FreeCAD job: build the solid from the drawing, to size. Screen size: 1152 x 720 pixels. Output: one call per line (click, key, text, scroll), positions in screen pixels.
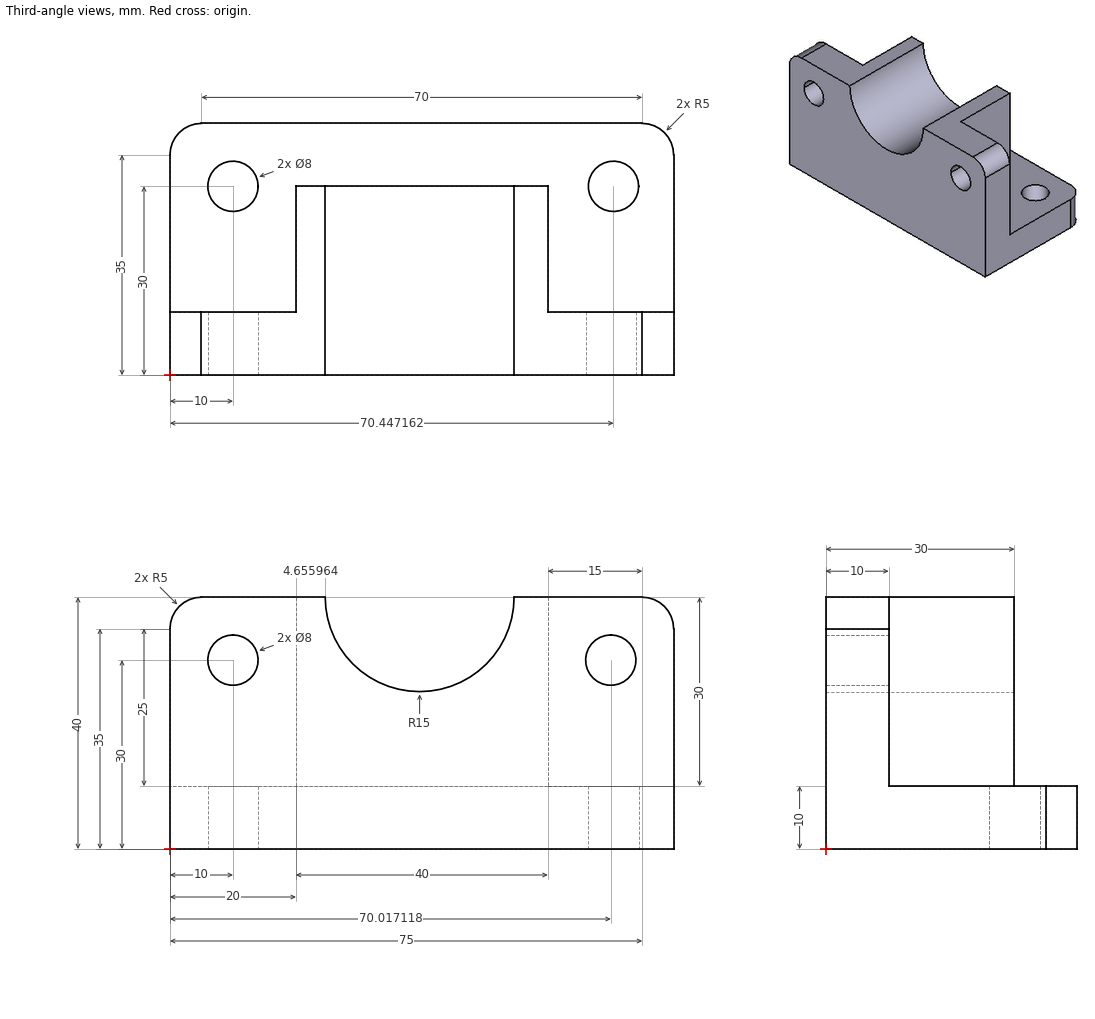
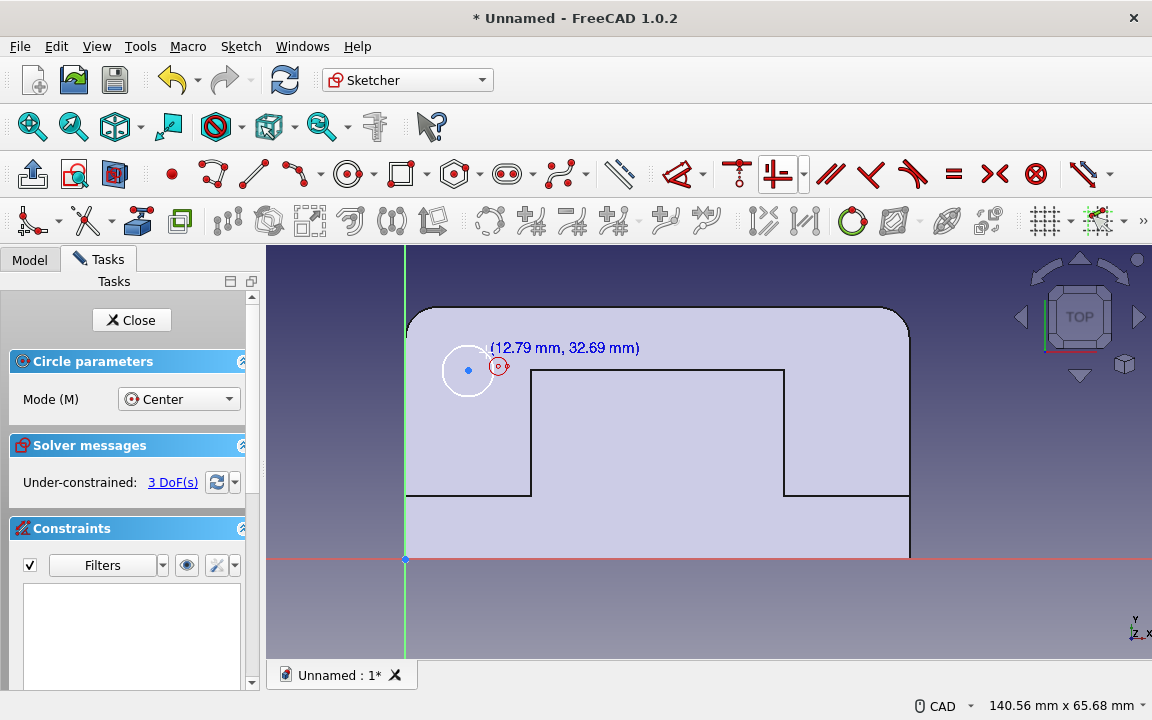
click(849, 370)
click(867, 352)
key(Escape)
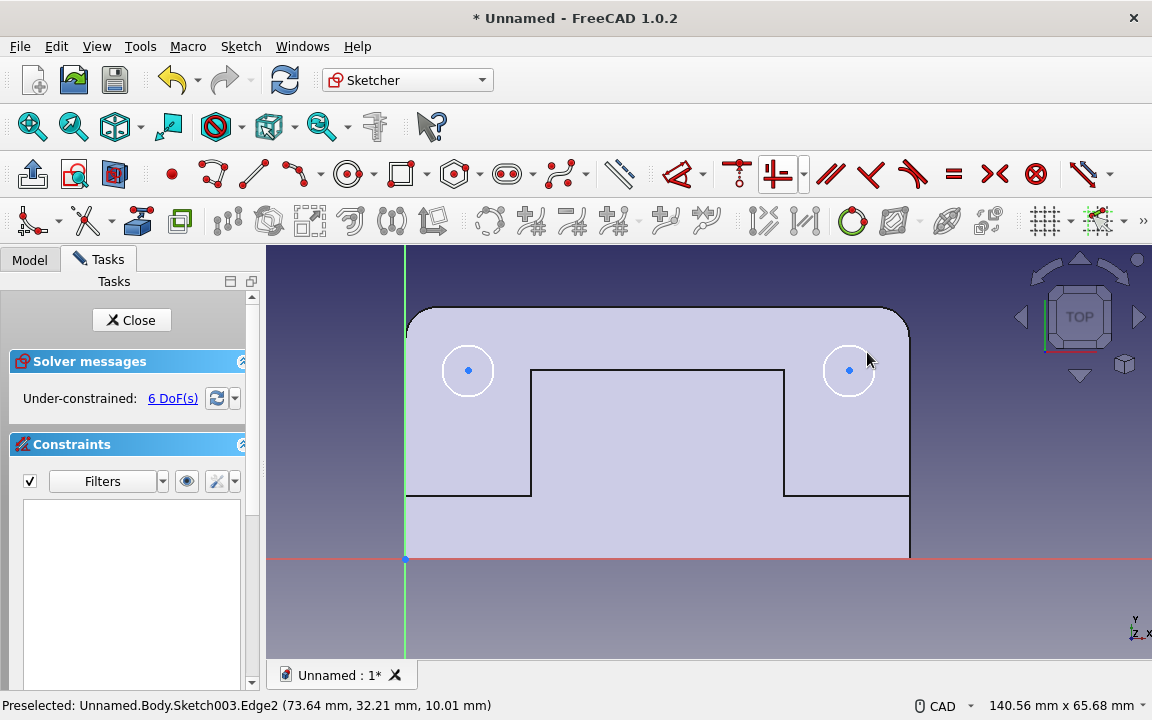
click(486, 353)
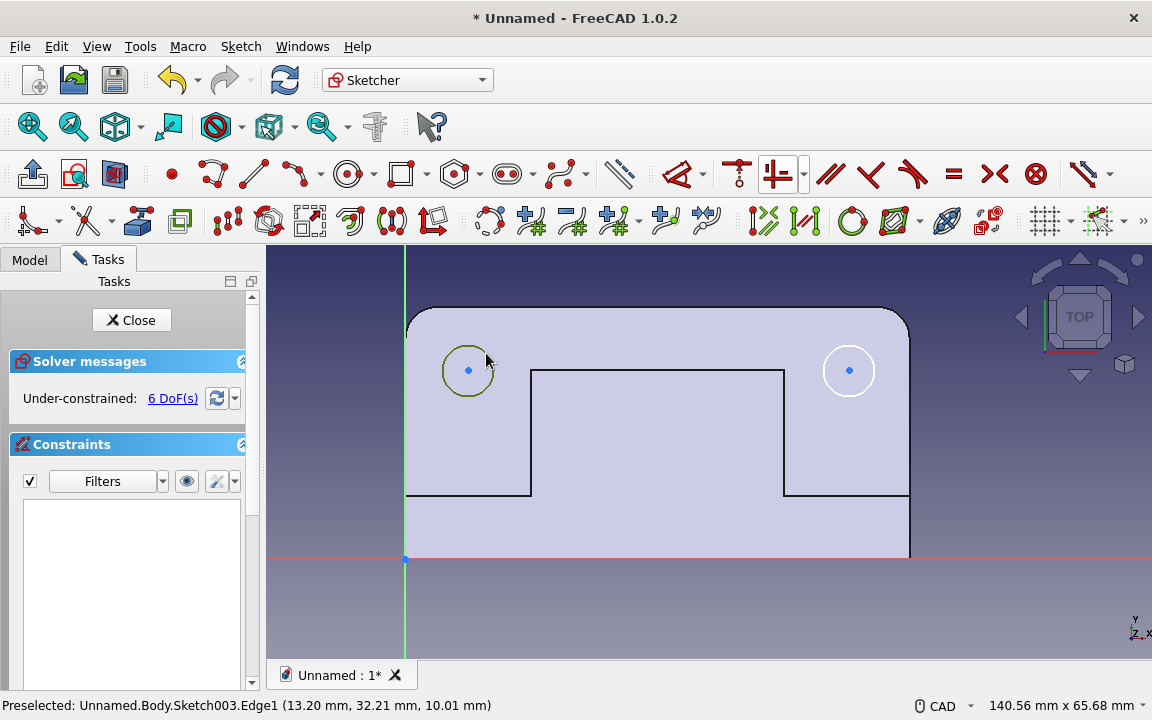
click(867, 353)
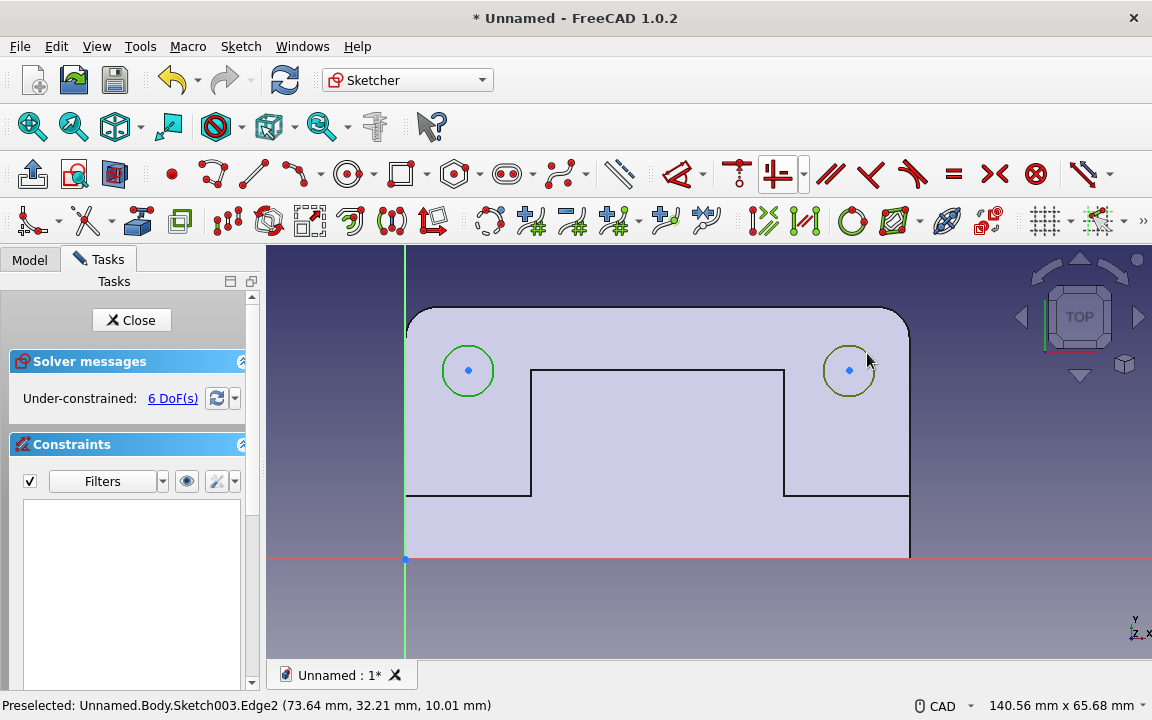
click(954, 174)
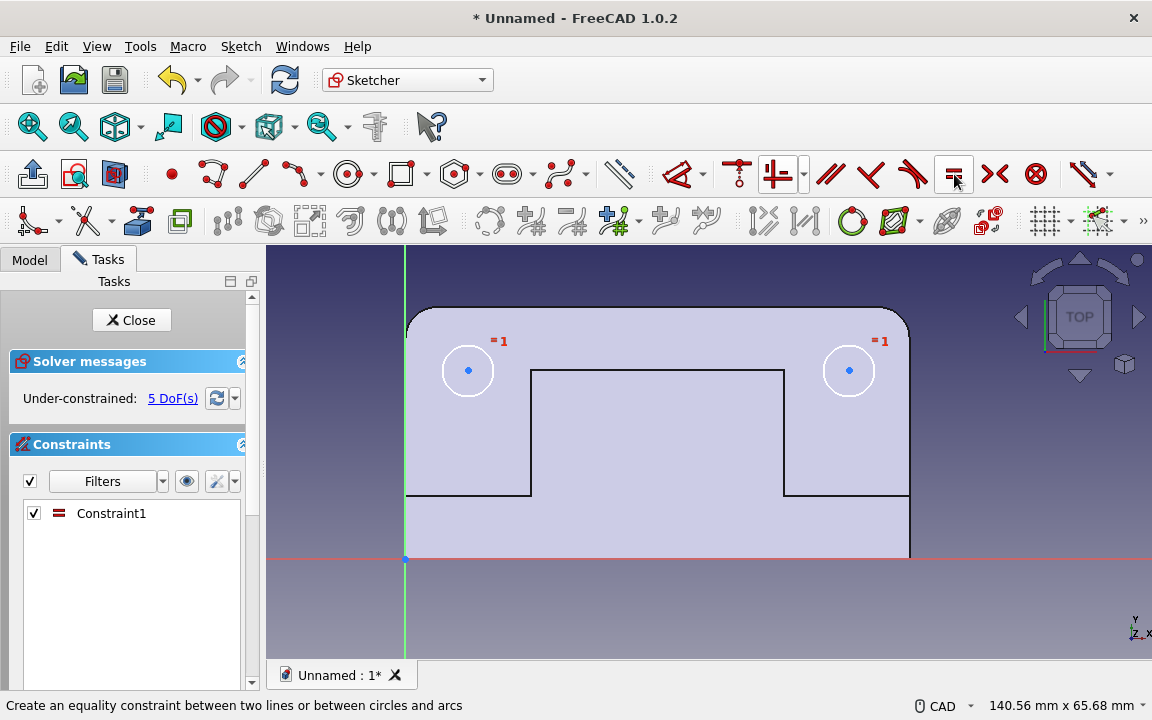
click(468, 371)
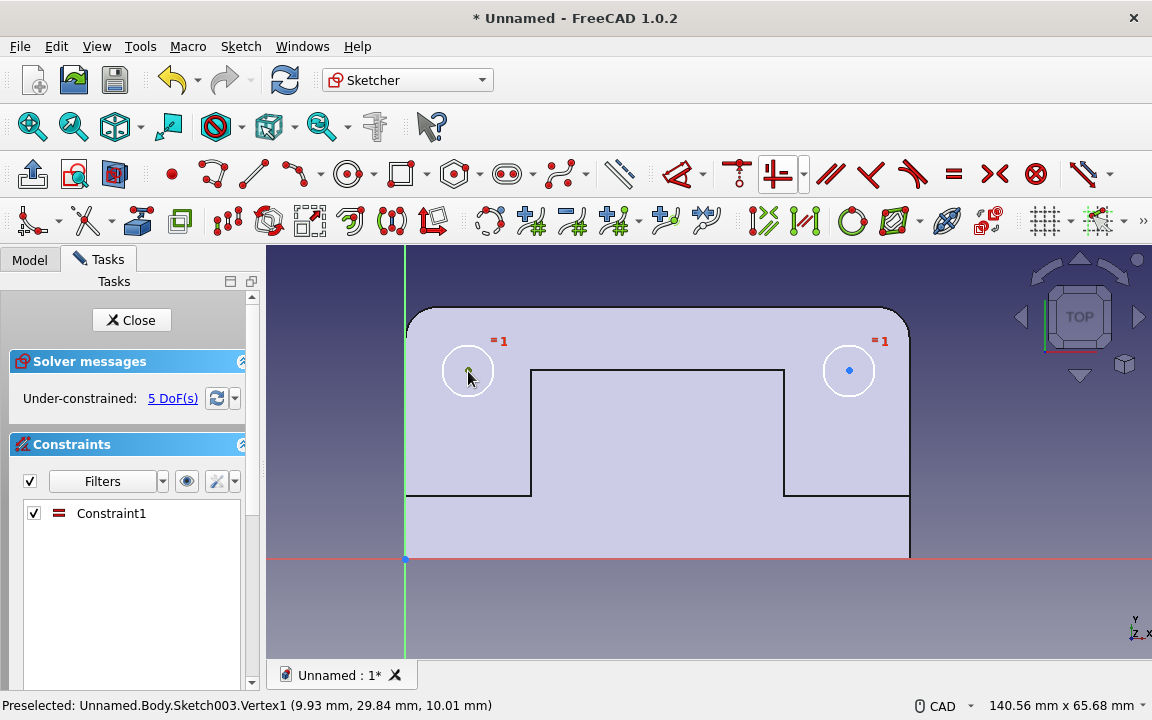
click(849, 371)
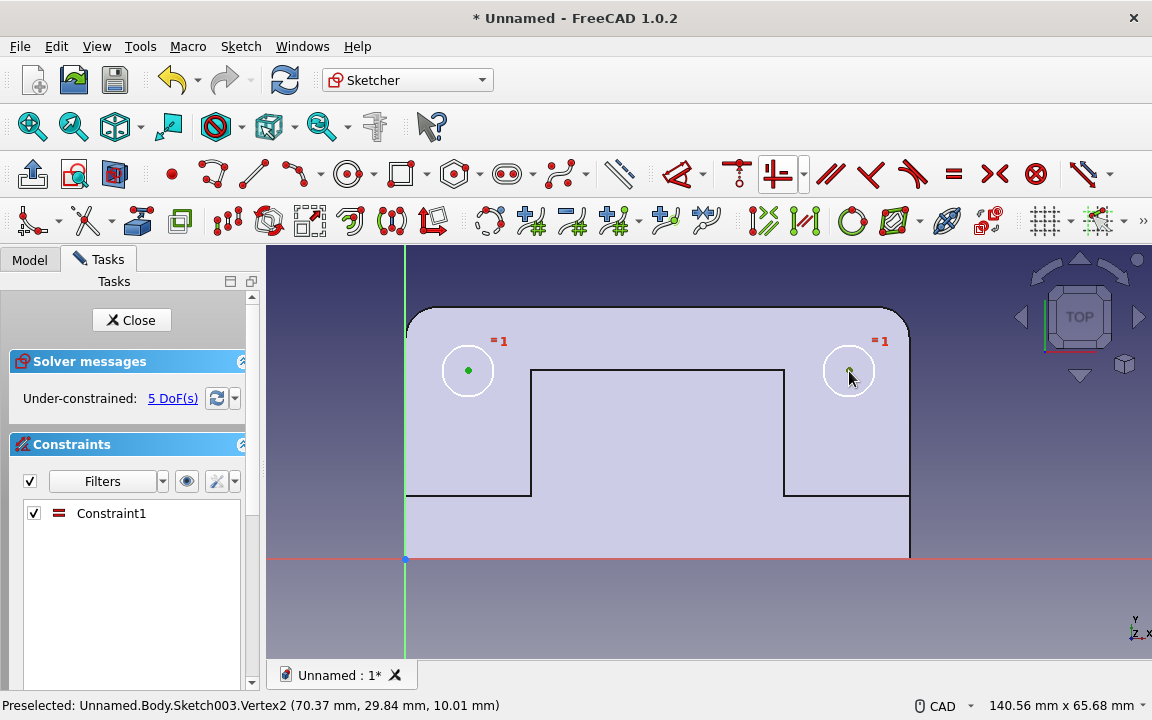
key(h)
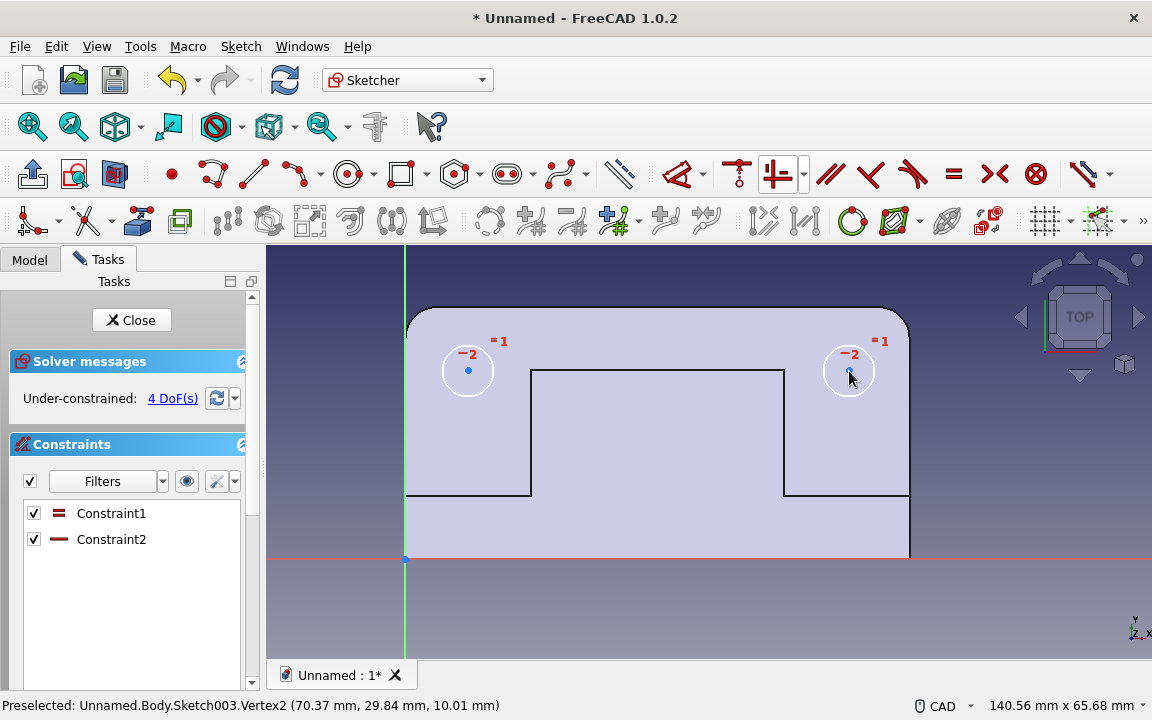
click(676, 174)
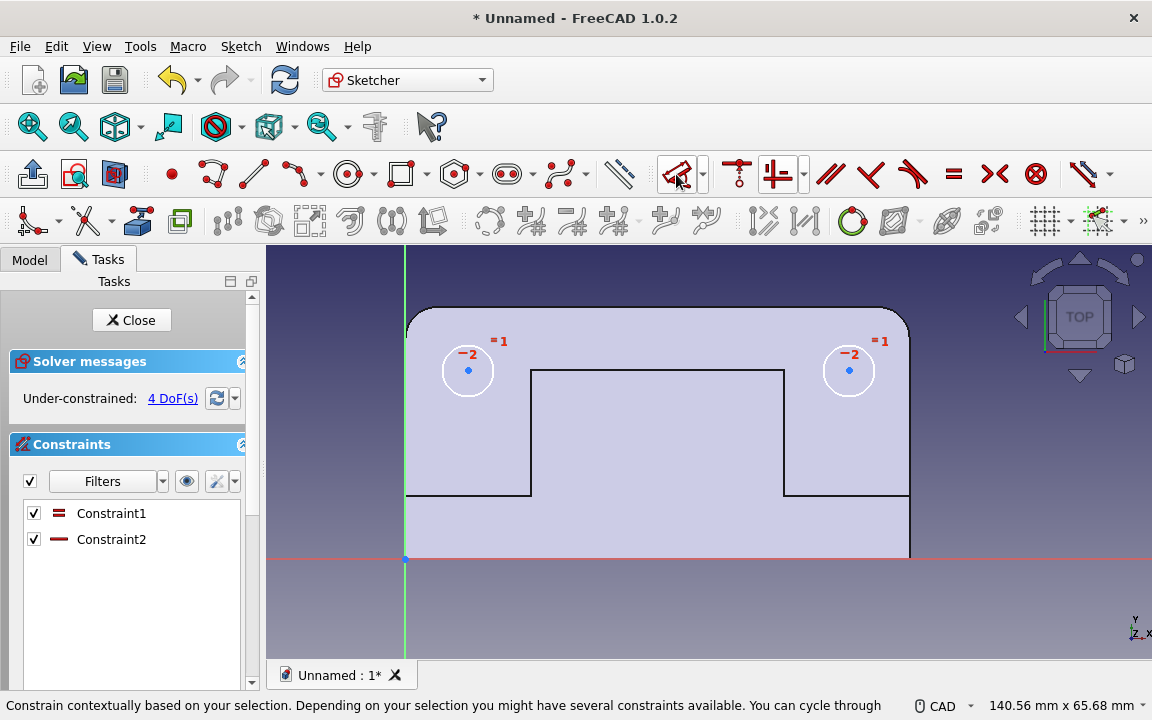
click(486, 353)
click(509, 330)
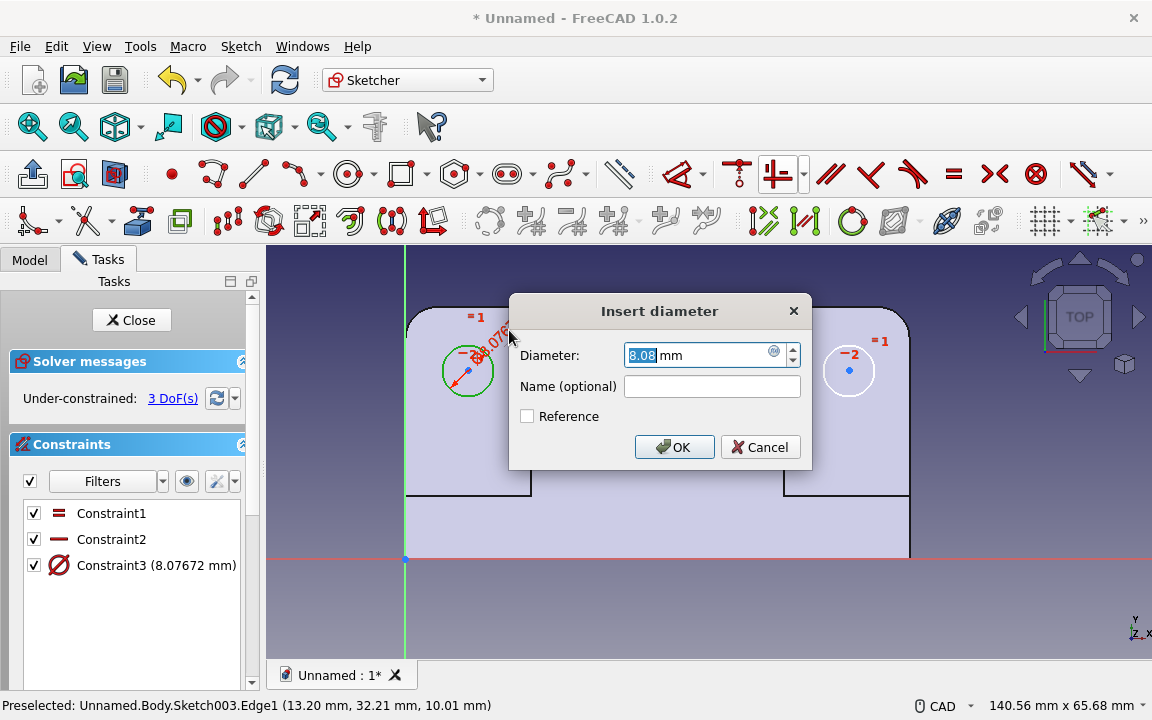
text(8)
key(Return)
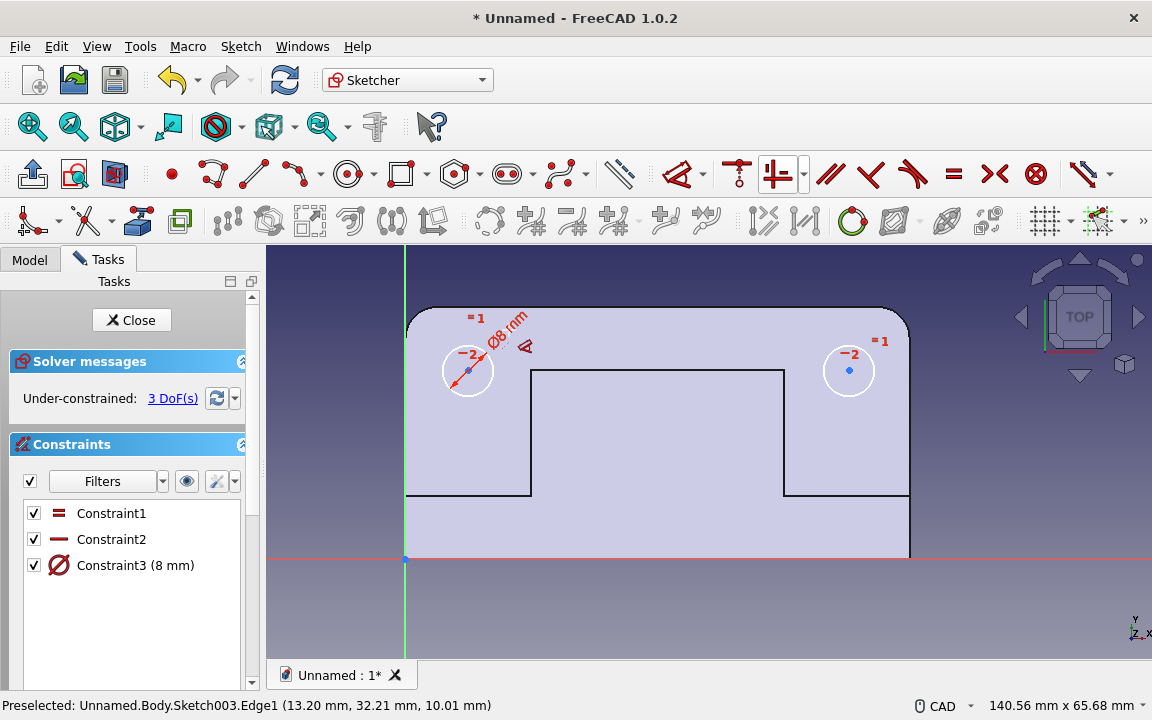
click(468, 371)
click(437, 593)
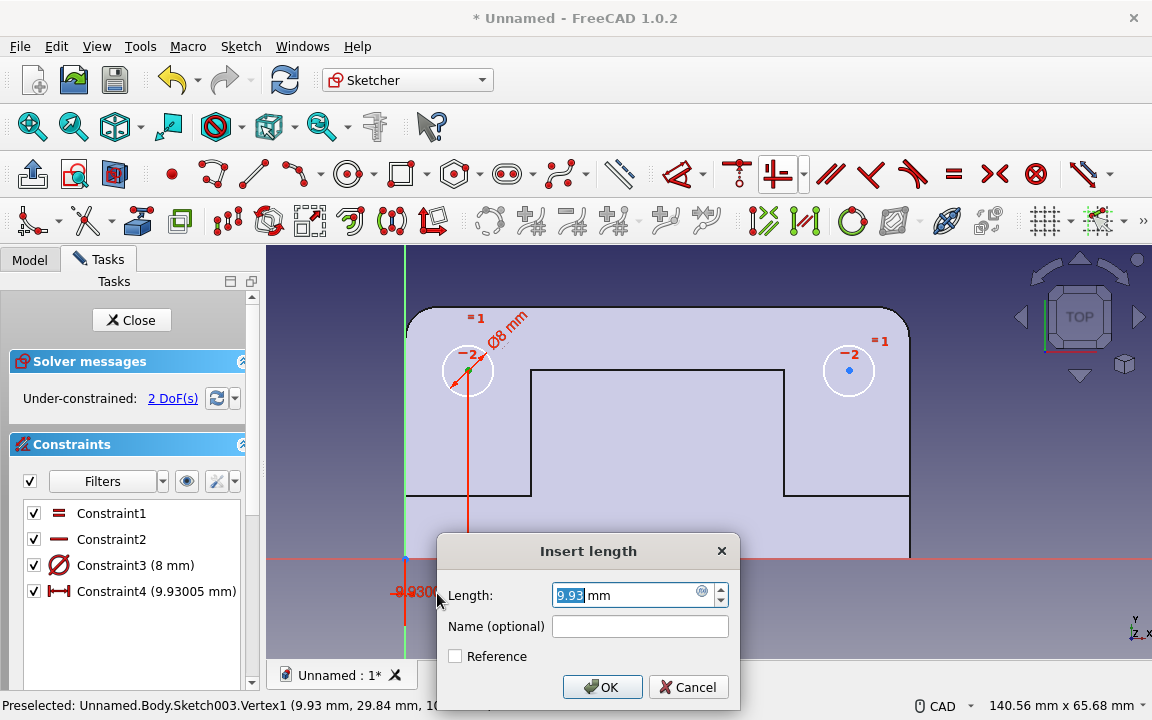
text(10)
key(Return)